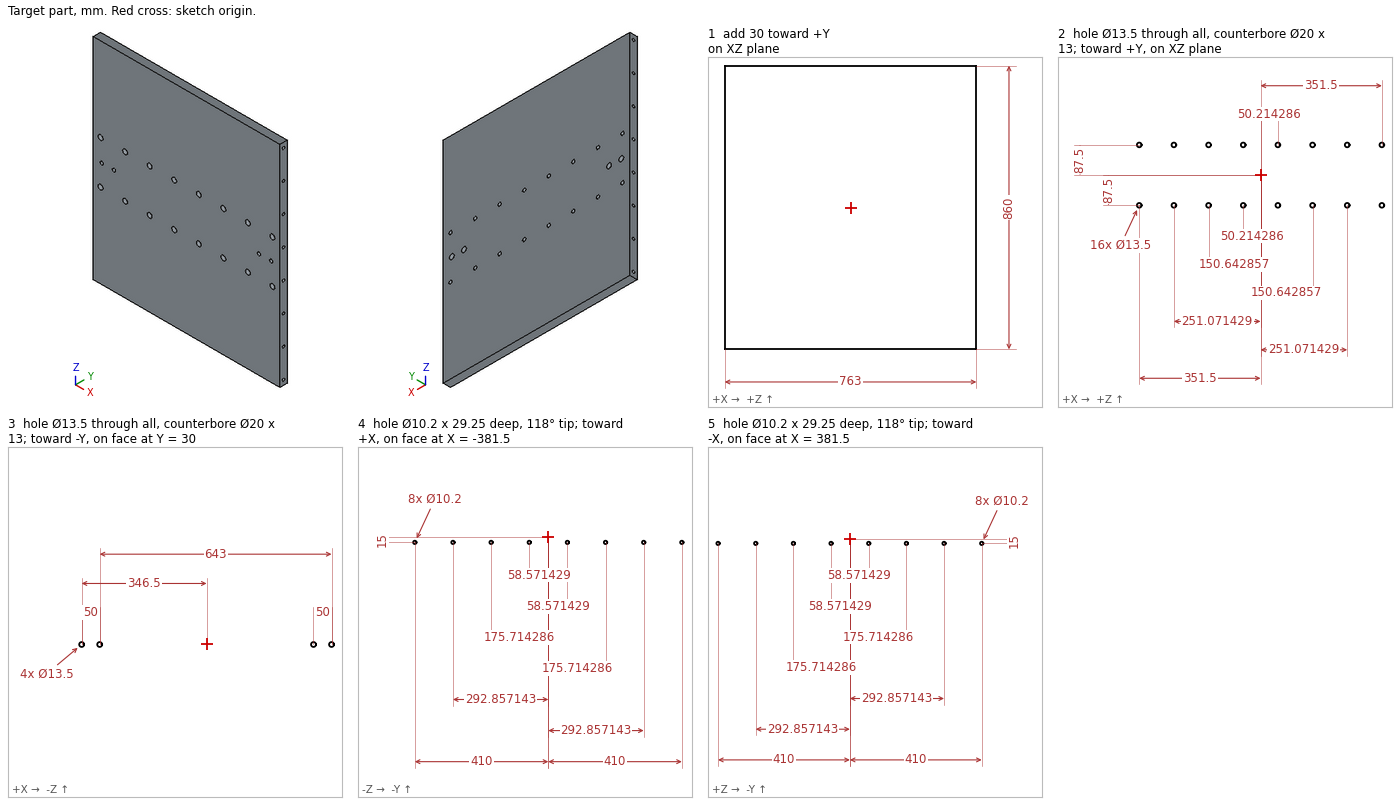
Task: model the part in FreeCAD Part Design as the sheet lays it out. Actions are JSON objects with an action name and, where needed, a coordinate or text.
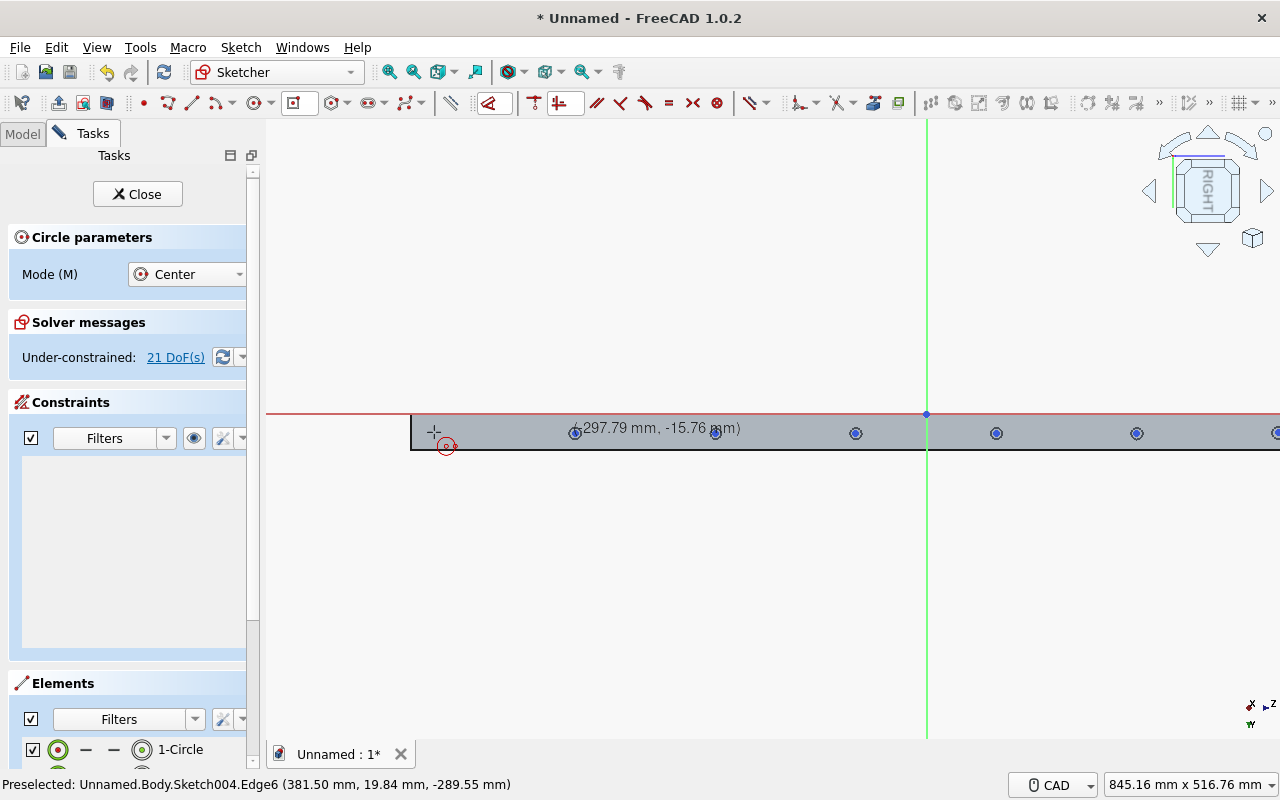
{"action": "left_click", "coordinate": [435, 432]}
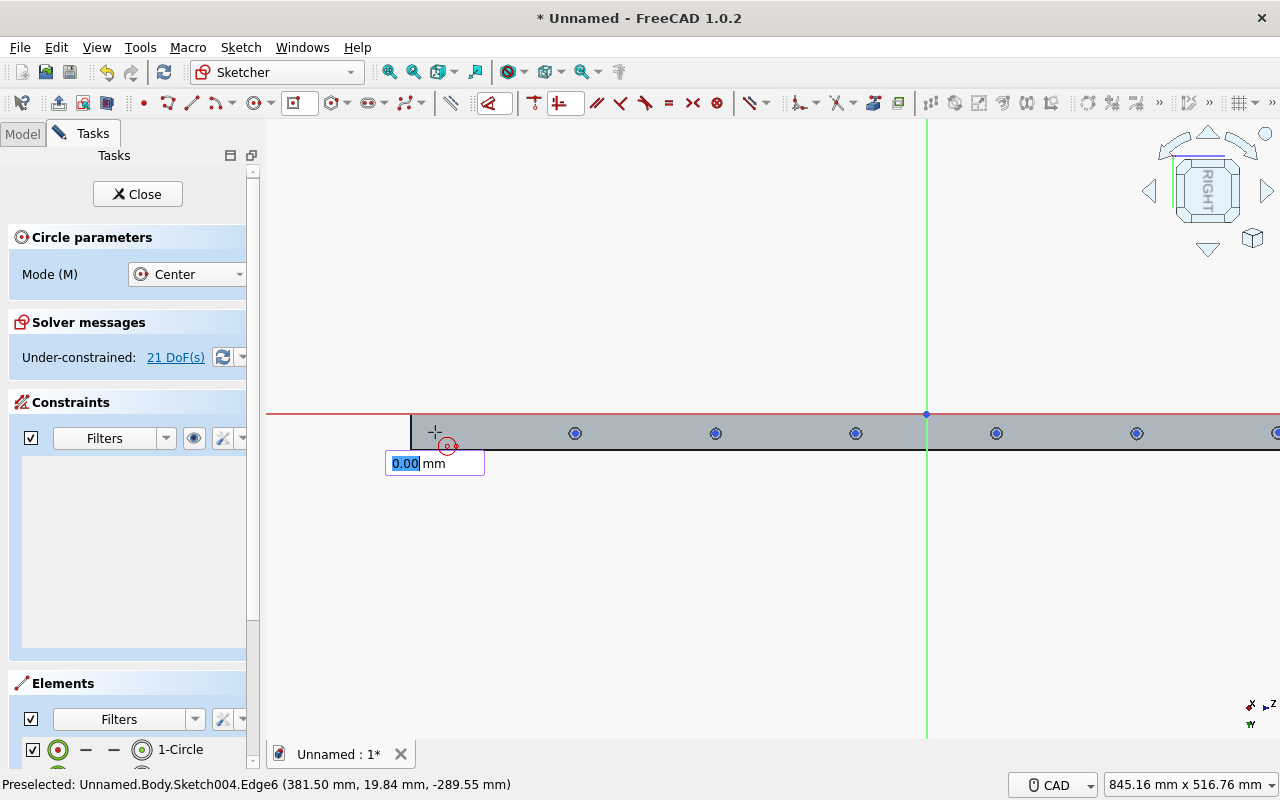
{"action": "scroll", "coordinate": [439, 437], "scroll_direction": "up", "scroll_amount": 5}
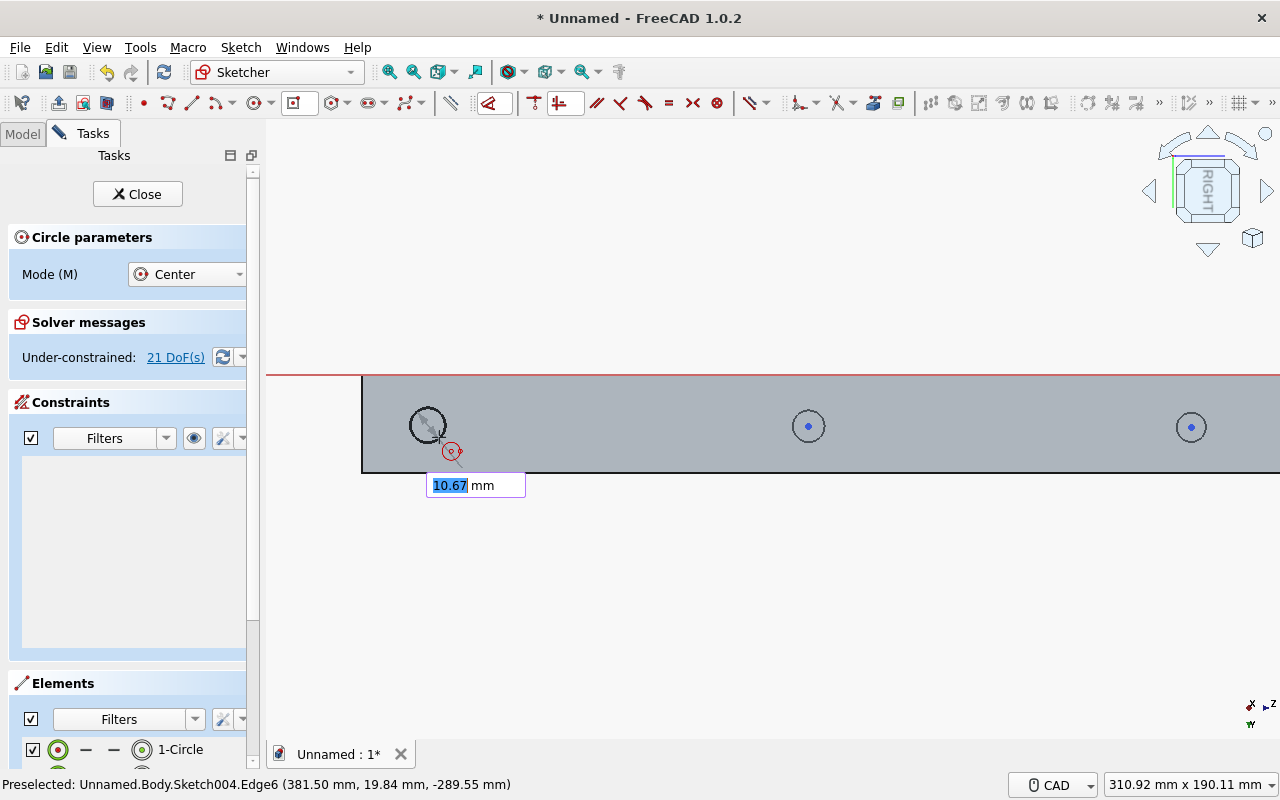
{"action": "left_click", "coordinate": [439, 436]}
{"action": "key", "text": "Escape"}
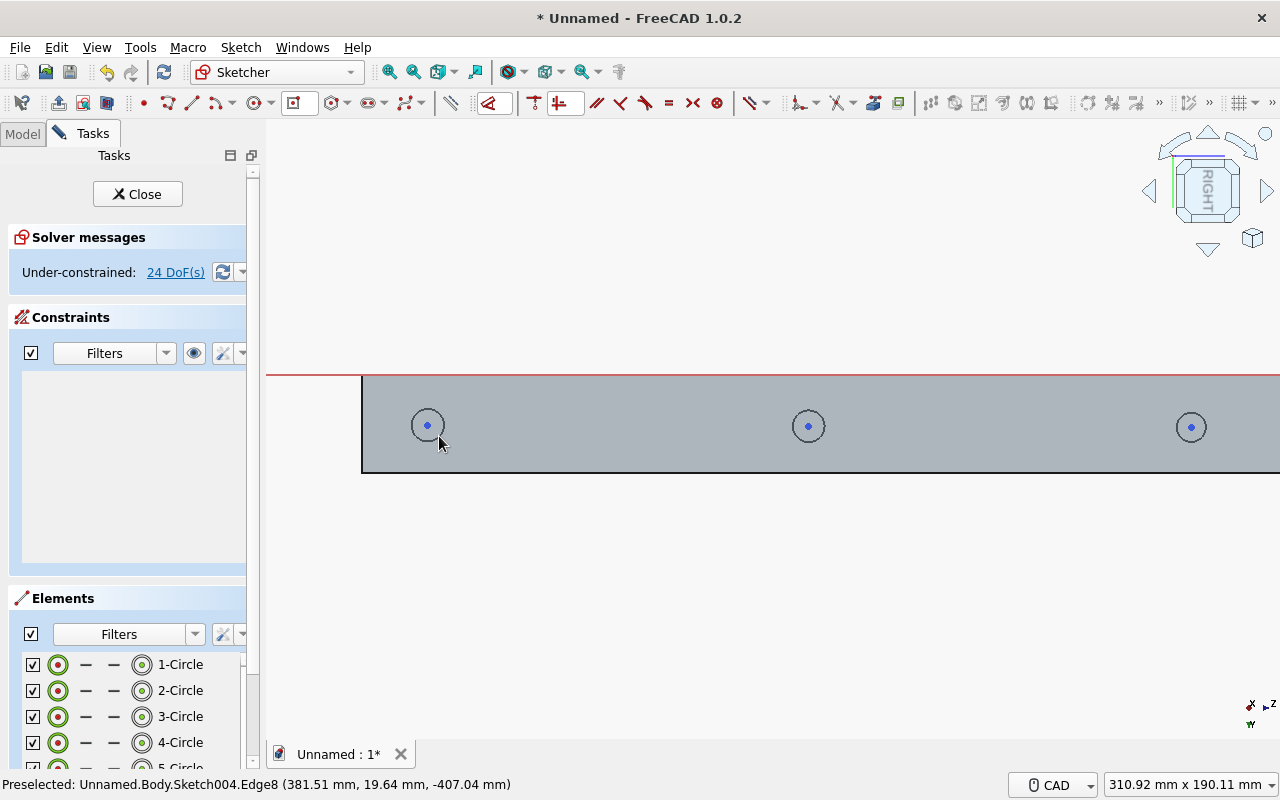
{"action": "scroll", "coordinate": [436, 434], "scroll_direction": "down", "scroll_amount": 8}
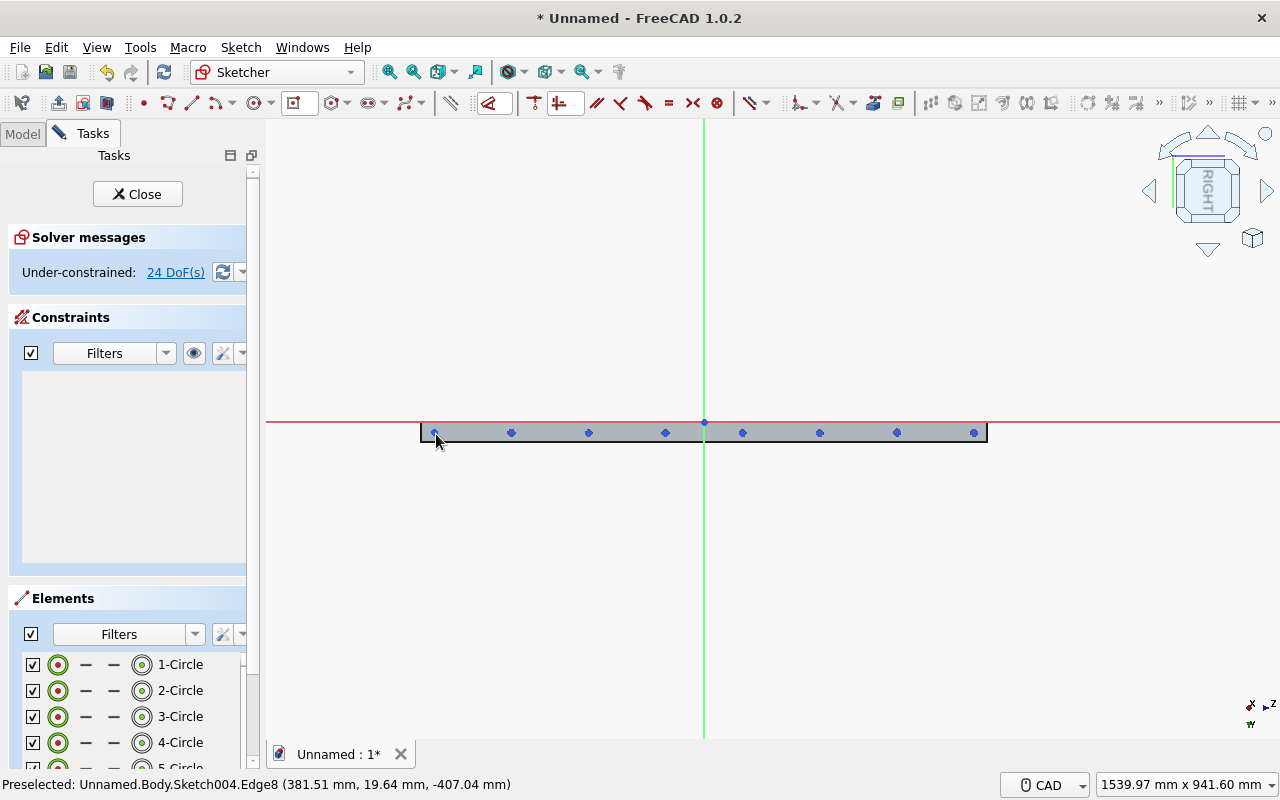
{"action": "scroll", "coordinate": [976, 430], "scroll_direction": "up", "scroll_amount": 8}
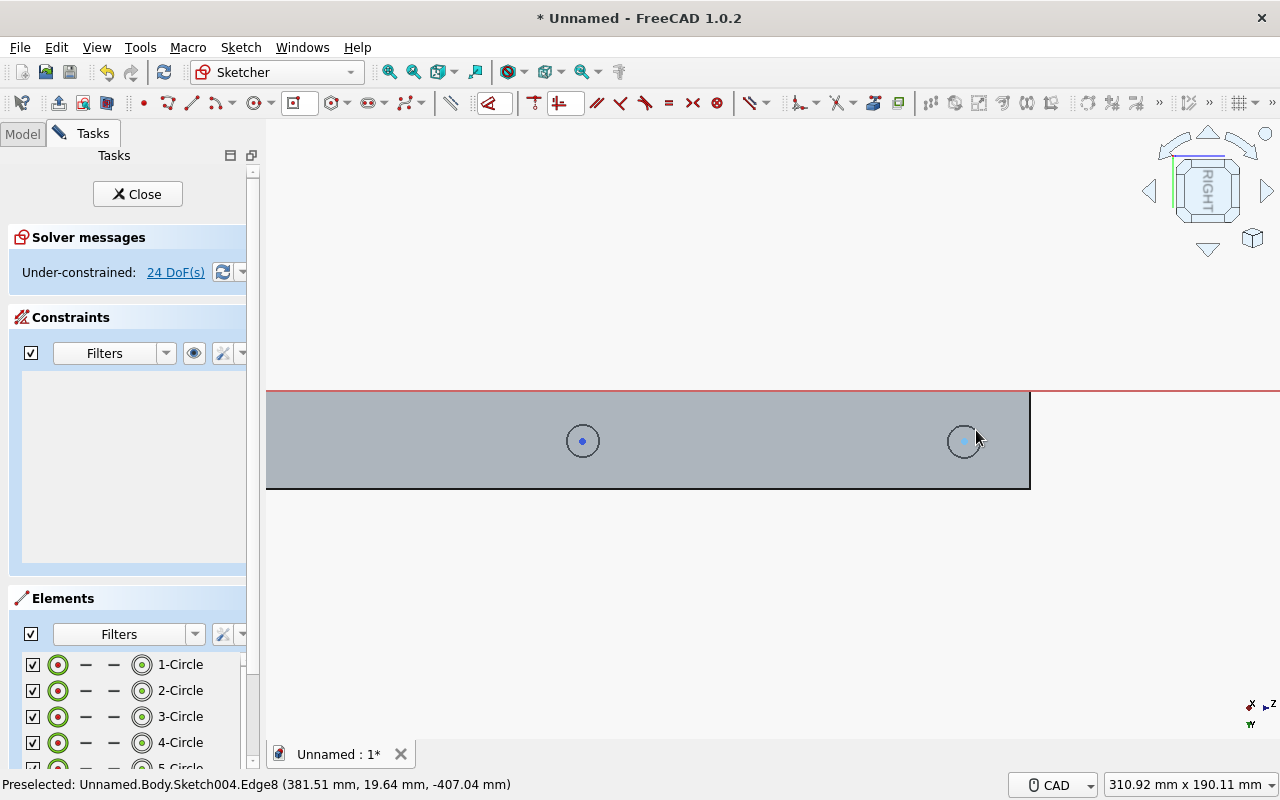
{"action": "left_click", "coordinate": [975, 430]}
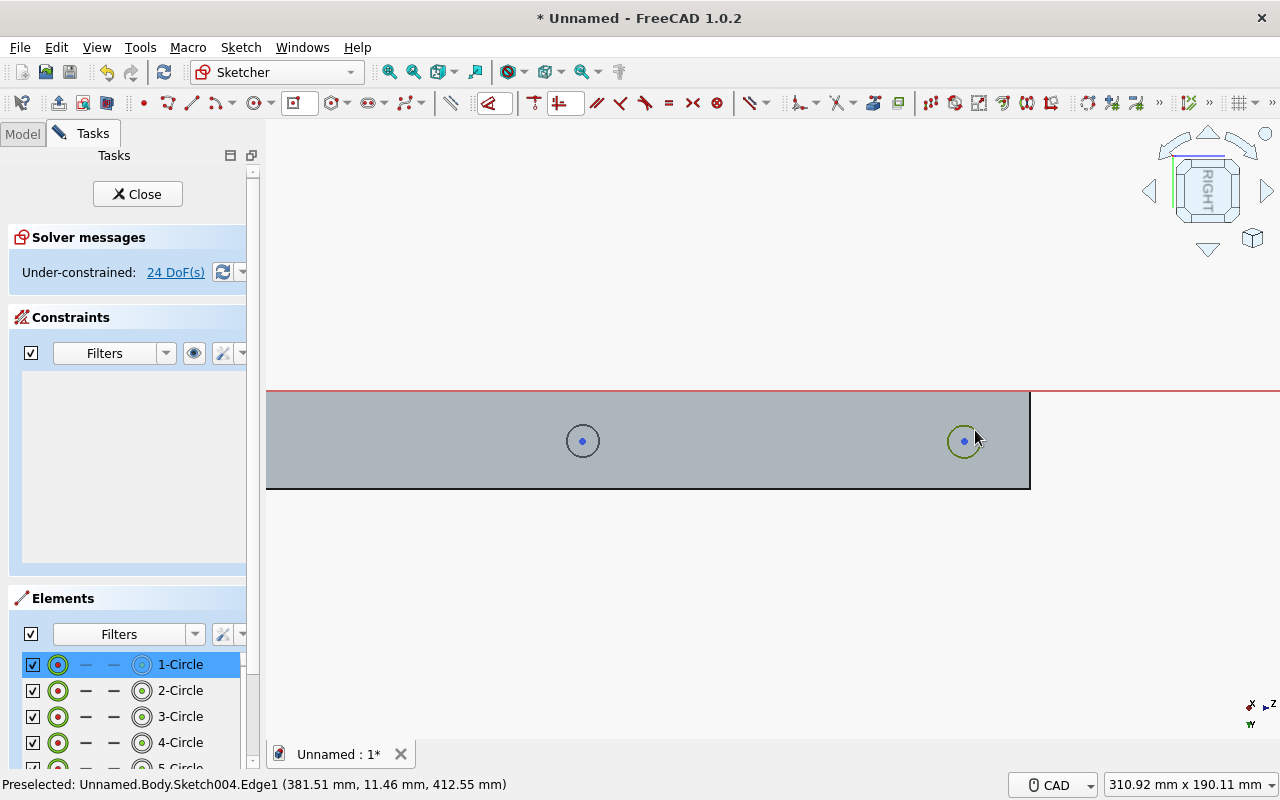
{"action": "left_click", "coordinate": [594, 430]}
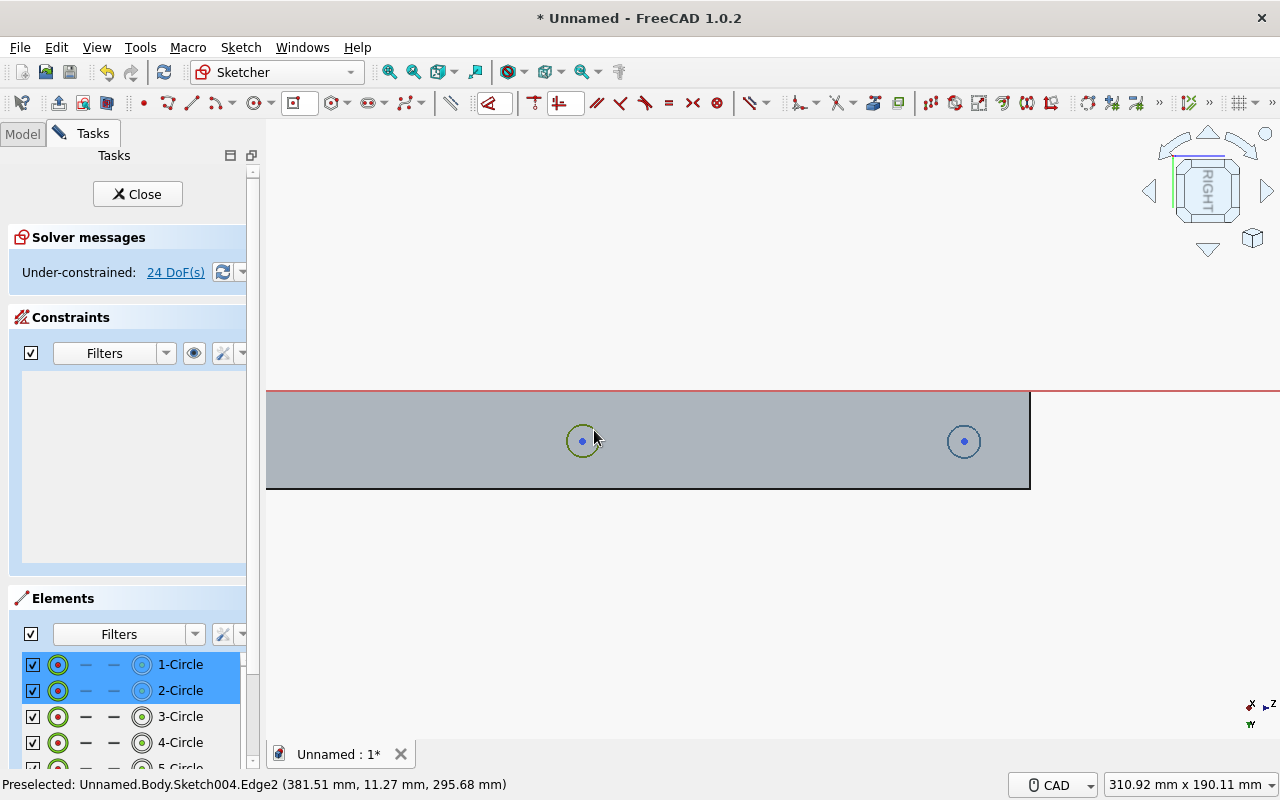
{"action": "scroll", "coordinate": [977, 430], "scroll_direction": "down", "scroll_amount": 8}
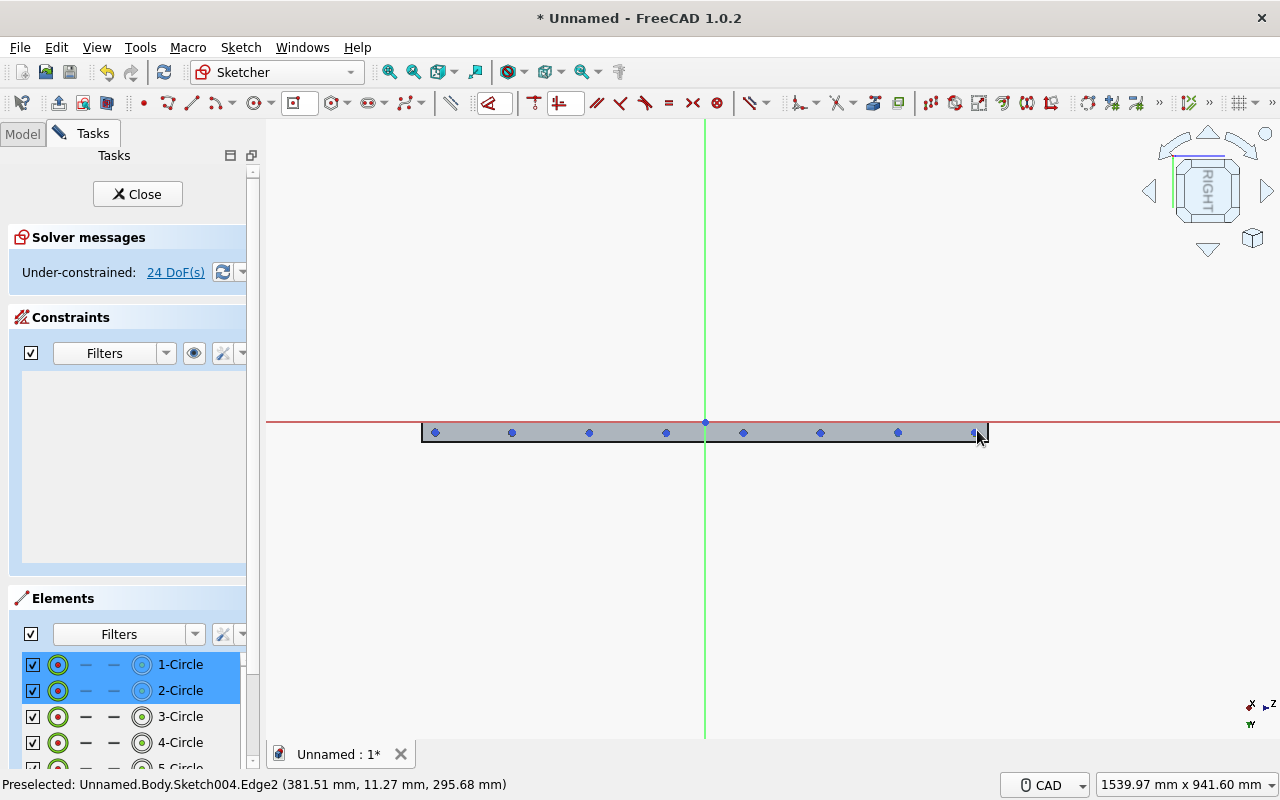
{"action": "scroll", "coordinate": [823, 431], "scroll_direction": "up", "scroll_amount": 8}